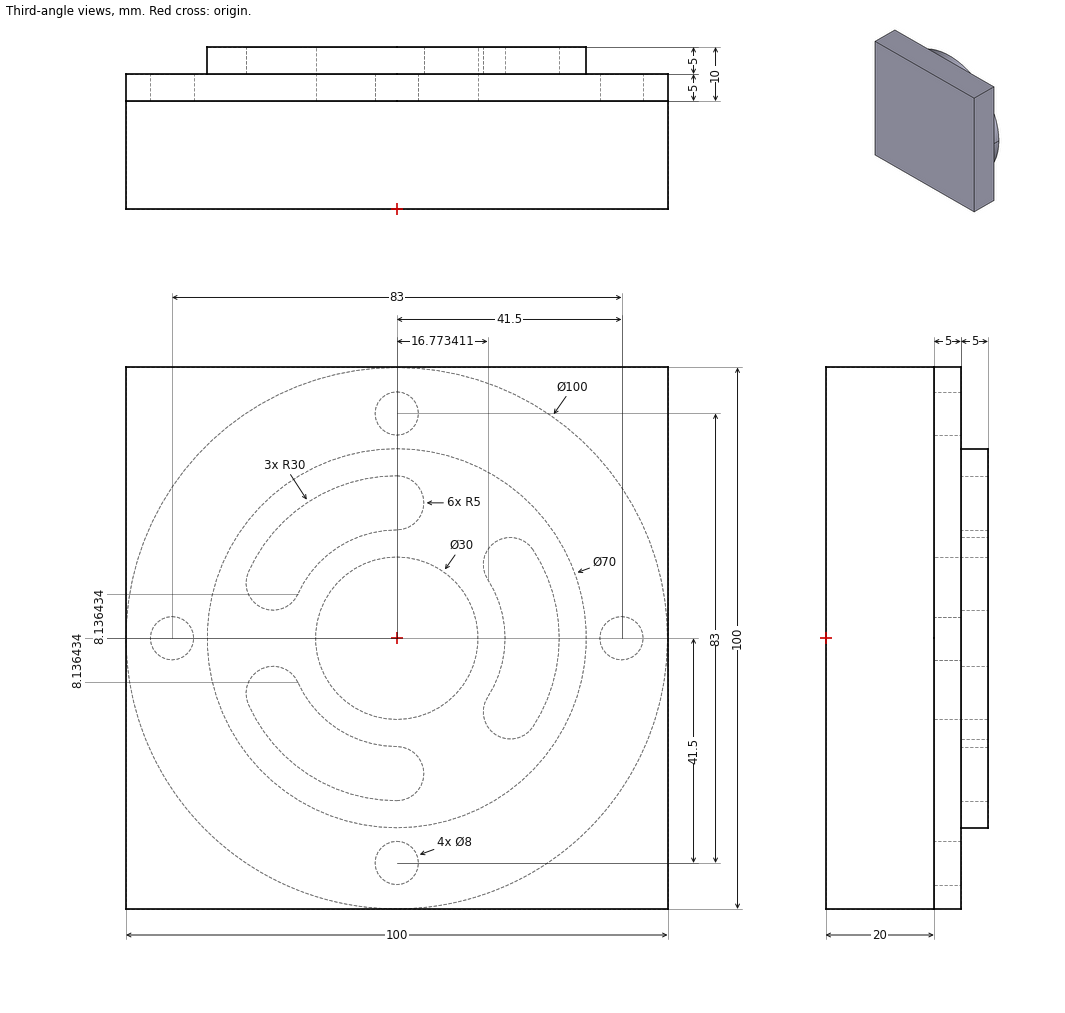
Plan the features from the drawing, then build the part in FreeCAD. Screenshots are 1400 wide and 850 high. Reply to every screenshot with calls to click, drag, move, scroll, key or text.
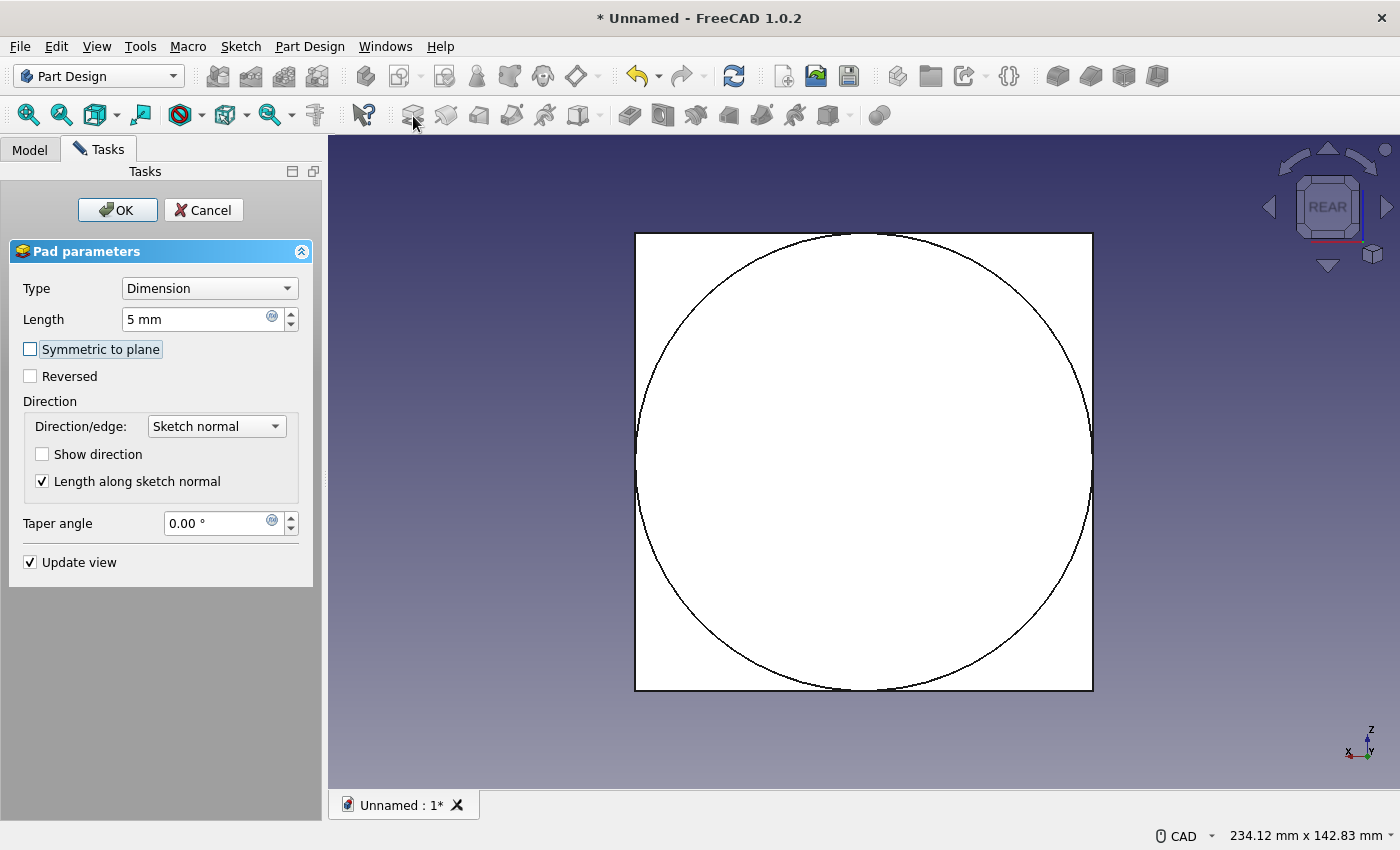
click(118, 210)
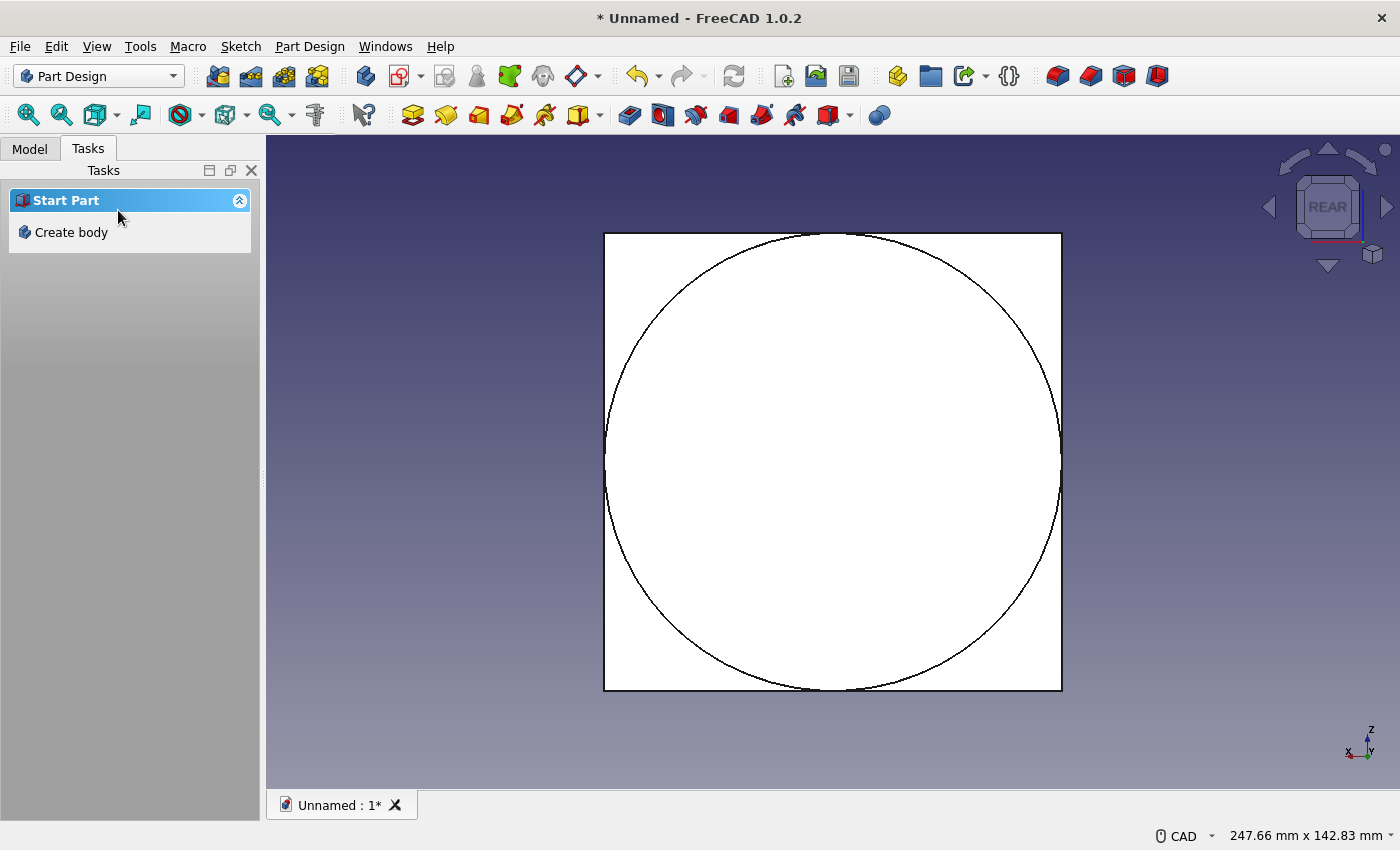
click(833, 461)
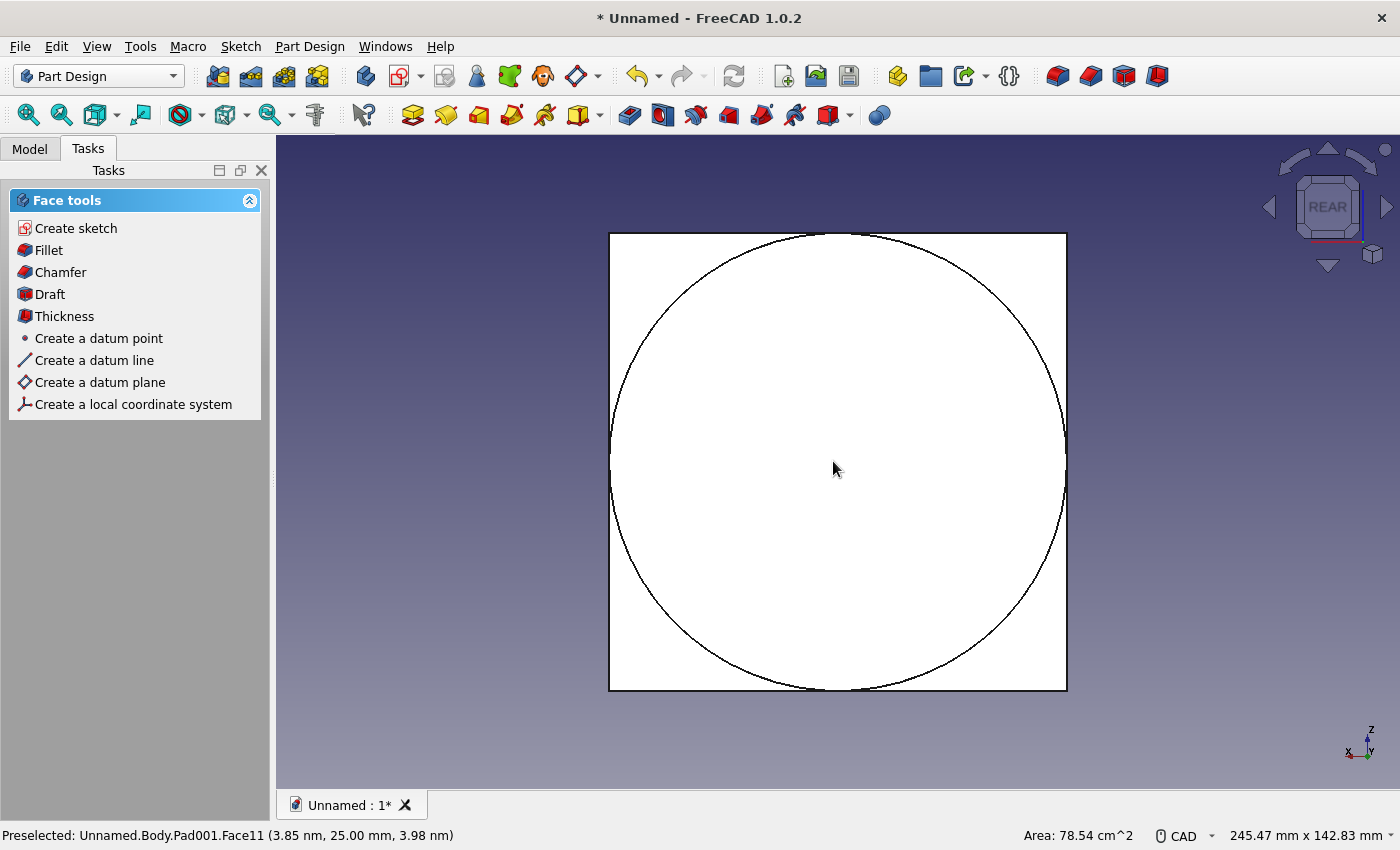
click(398, 76)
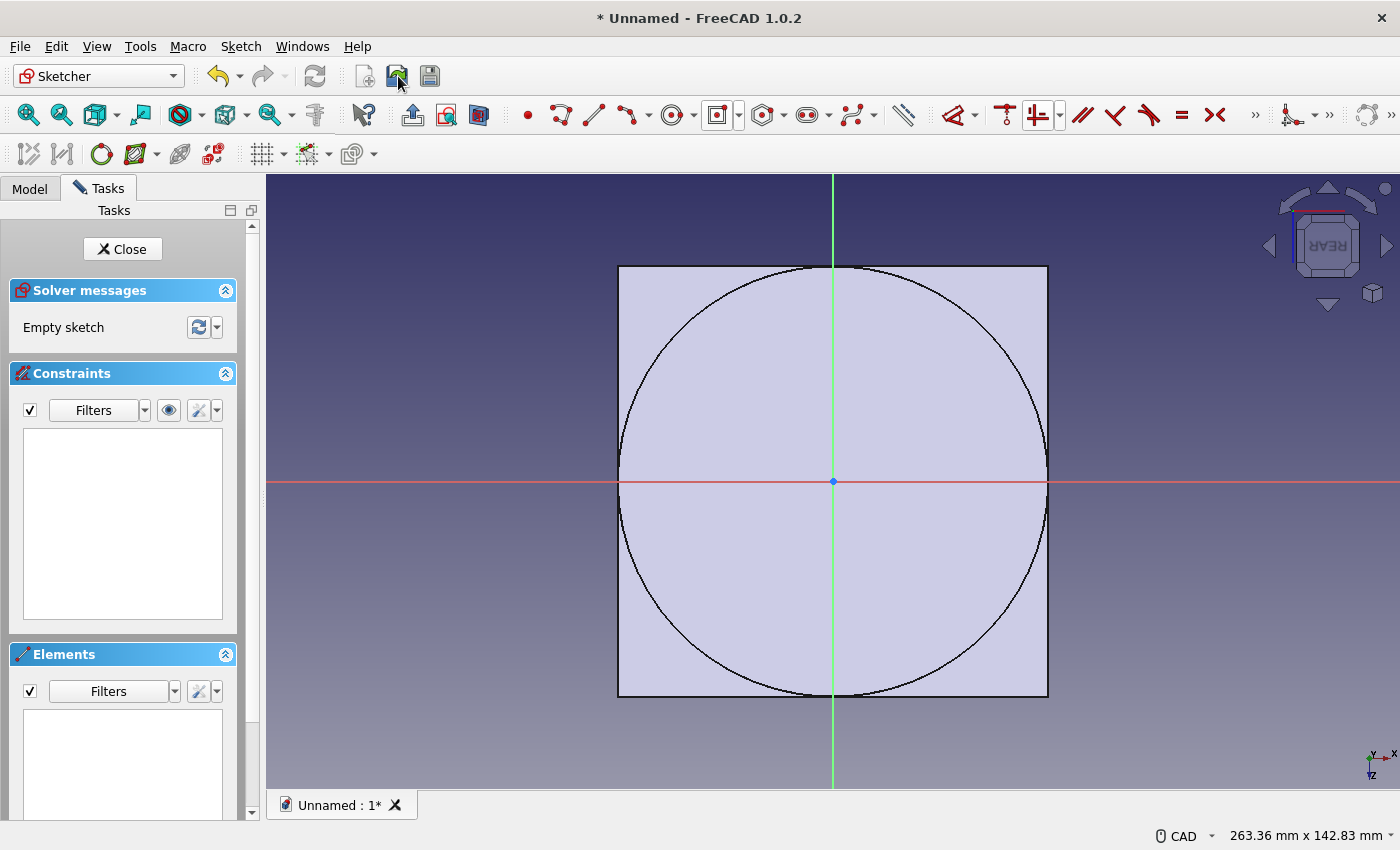
click(672, 116)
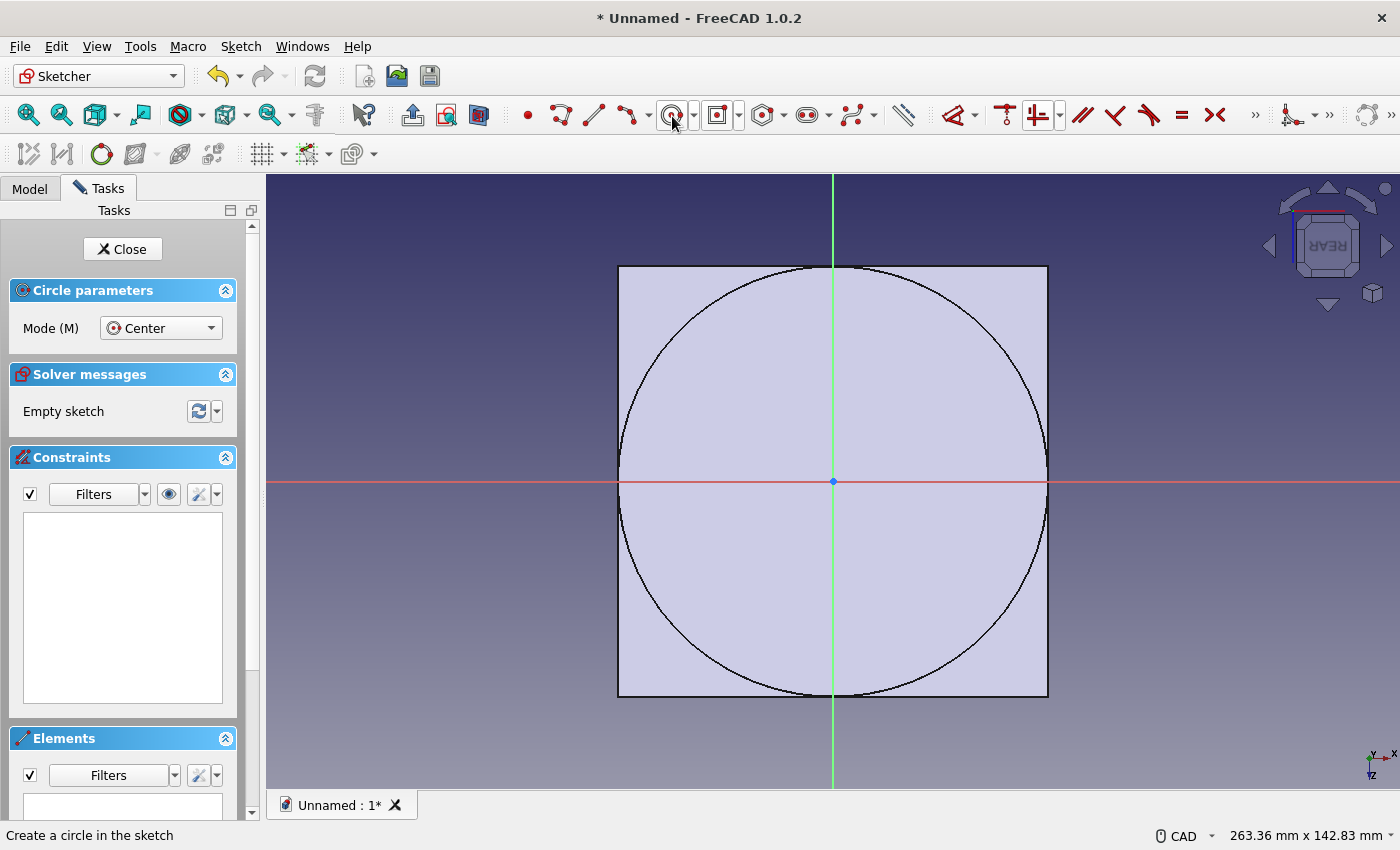
scroll(833, 303, up, 2)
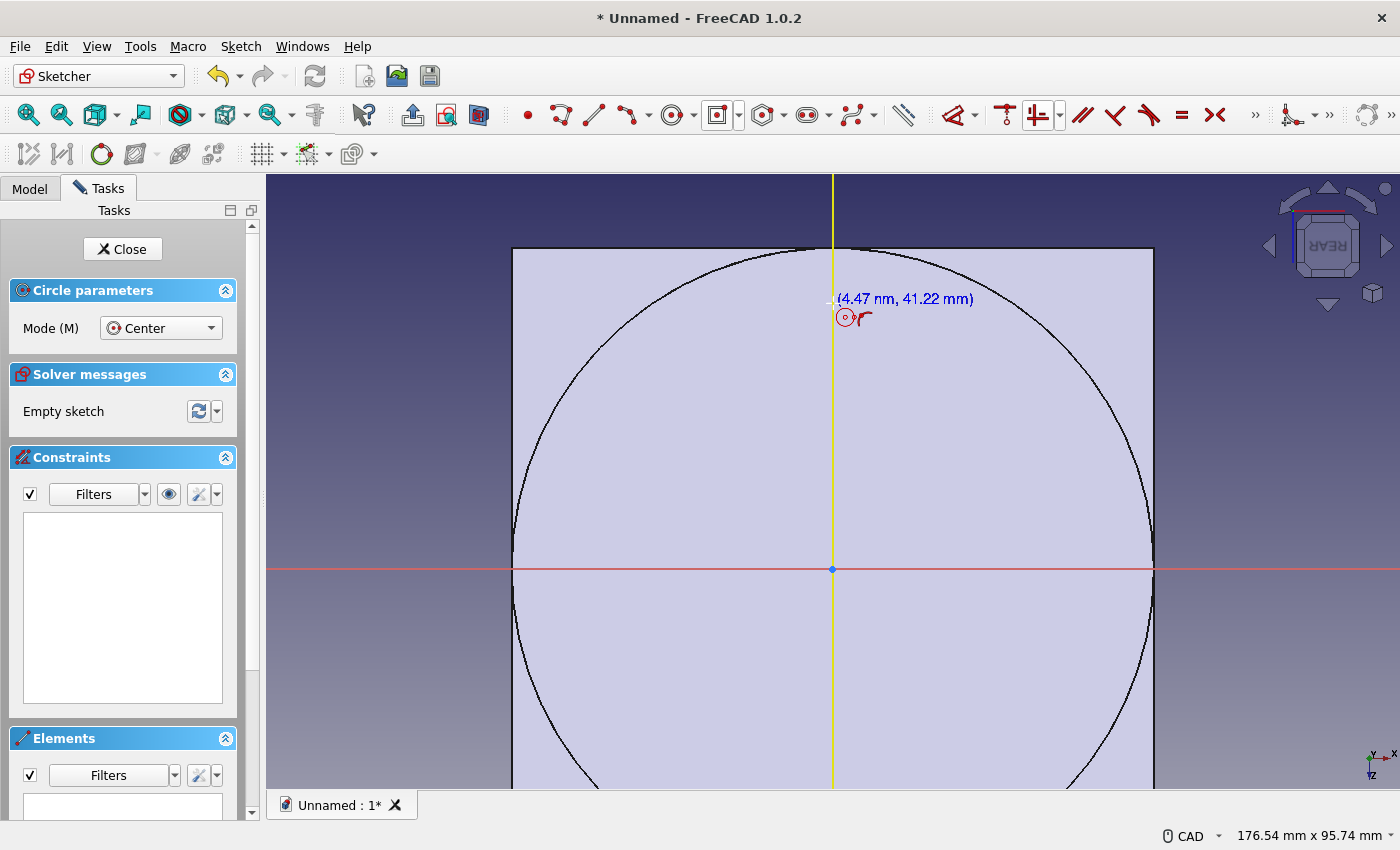
click(833, 303)
move(851, 284)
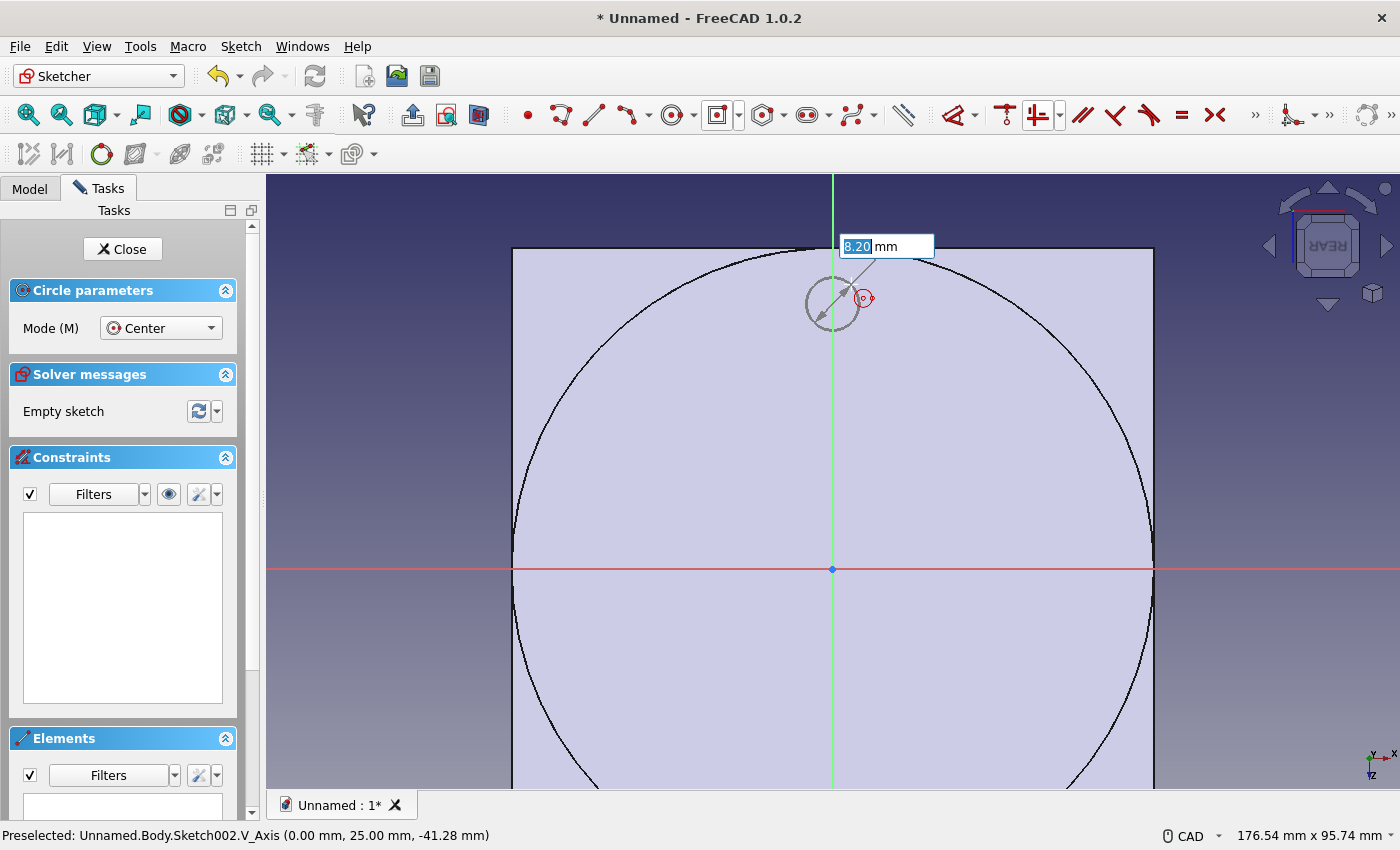
text(8)
key(Return)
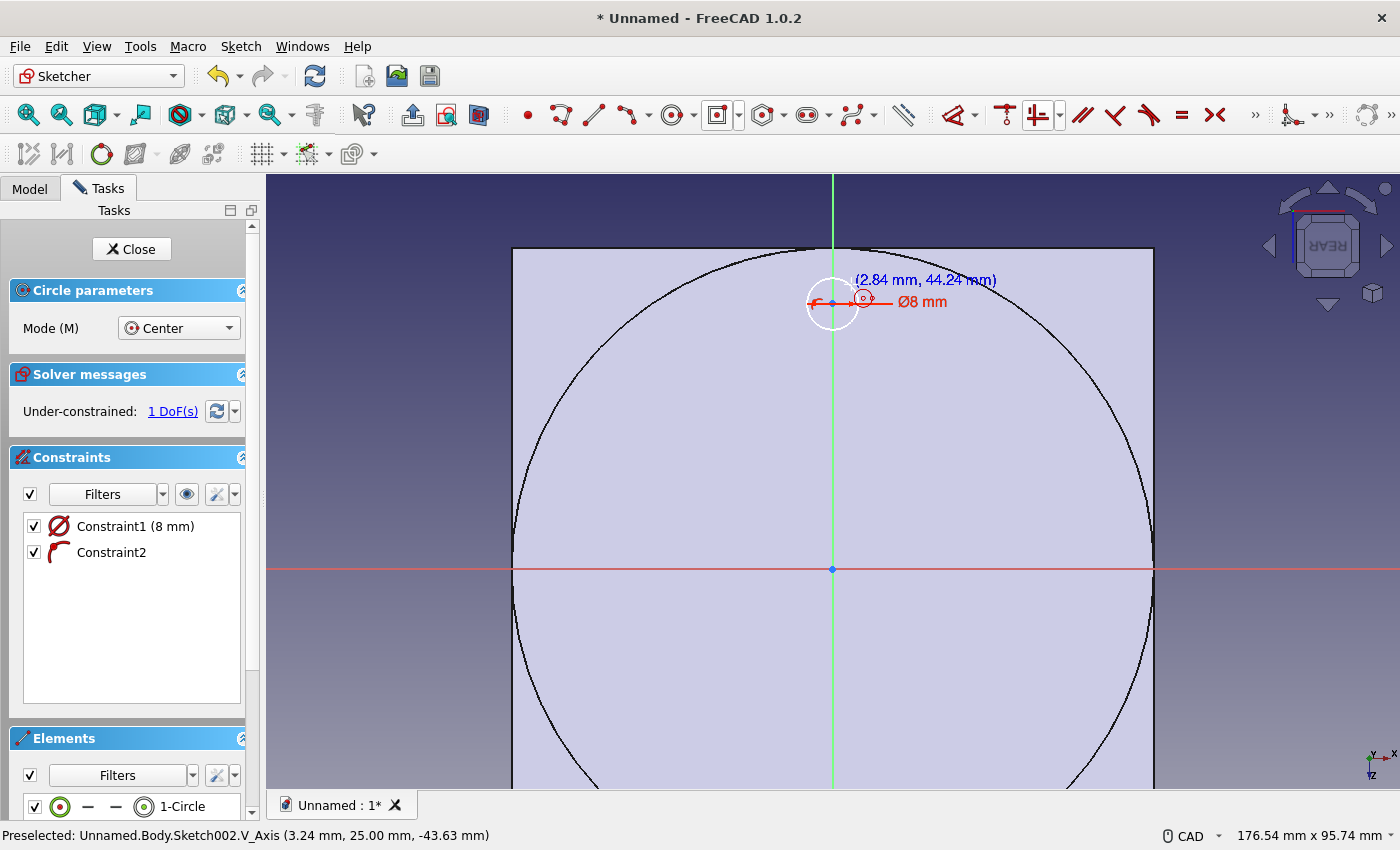
click(1099, 569)
move(1118, 551)